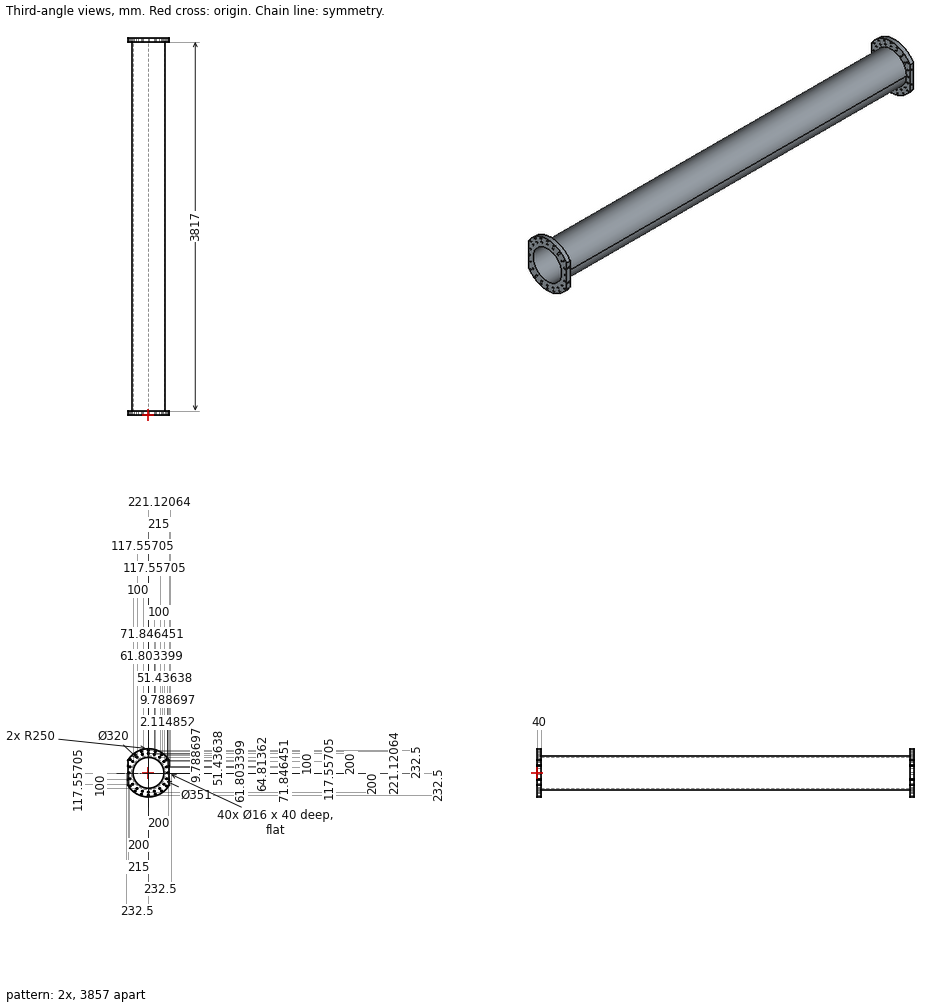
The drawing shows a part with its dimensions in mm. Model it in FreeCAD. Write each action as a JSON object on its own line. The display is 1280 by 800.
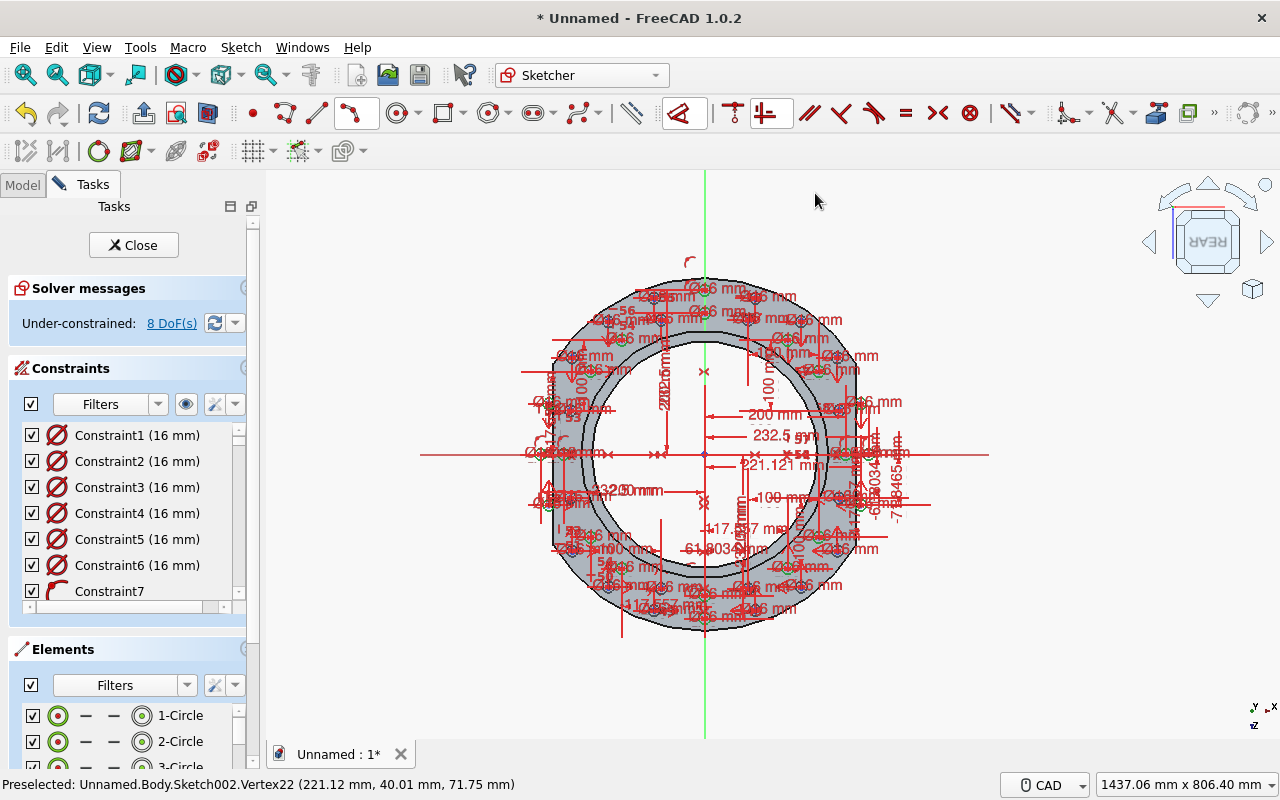
{"action": "left_click", "coordinate": [755, 611]}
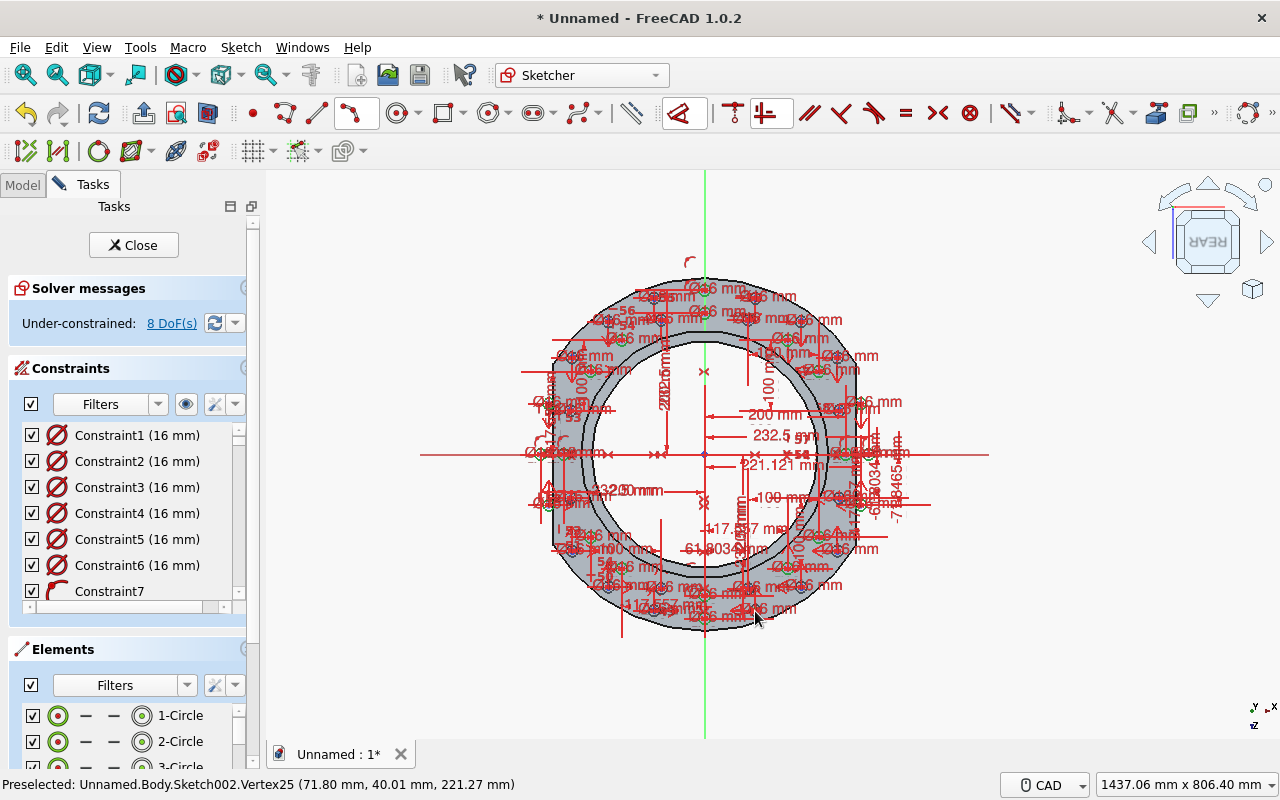
{"action": "left_click", "coordinate": [702, 114]}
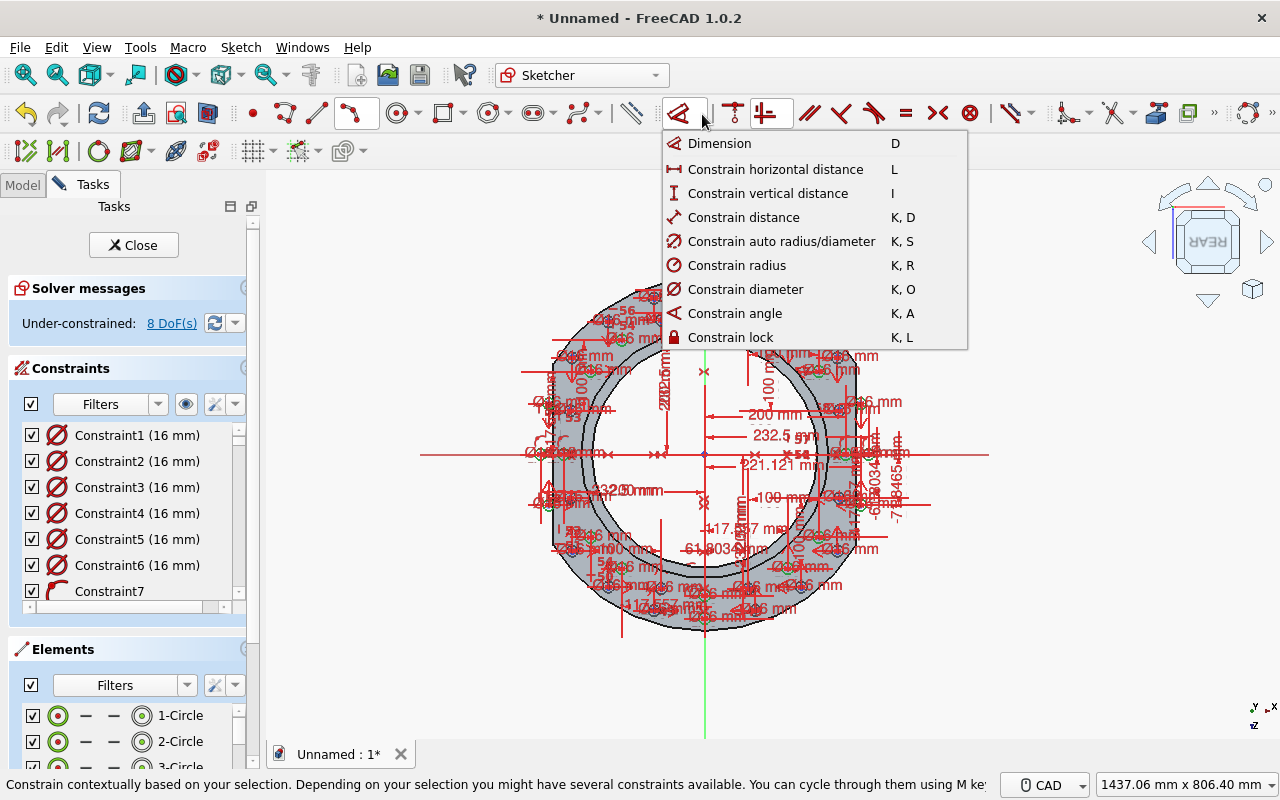
{"action": "left_click", "coordinate": [815, 169]}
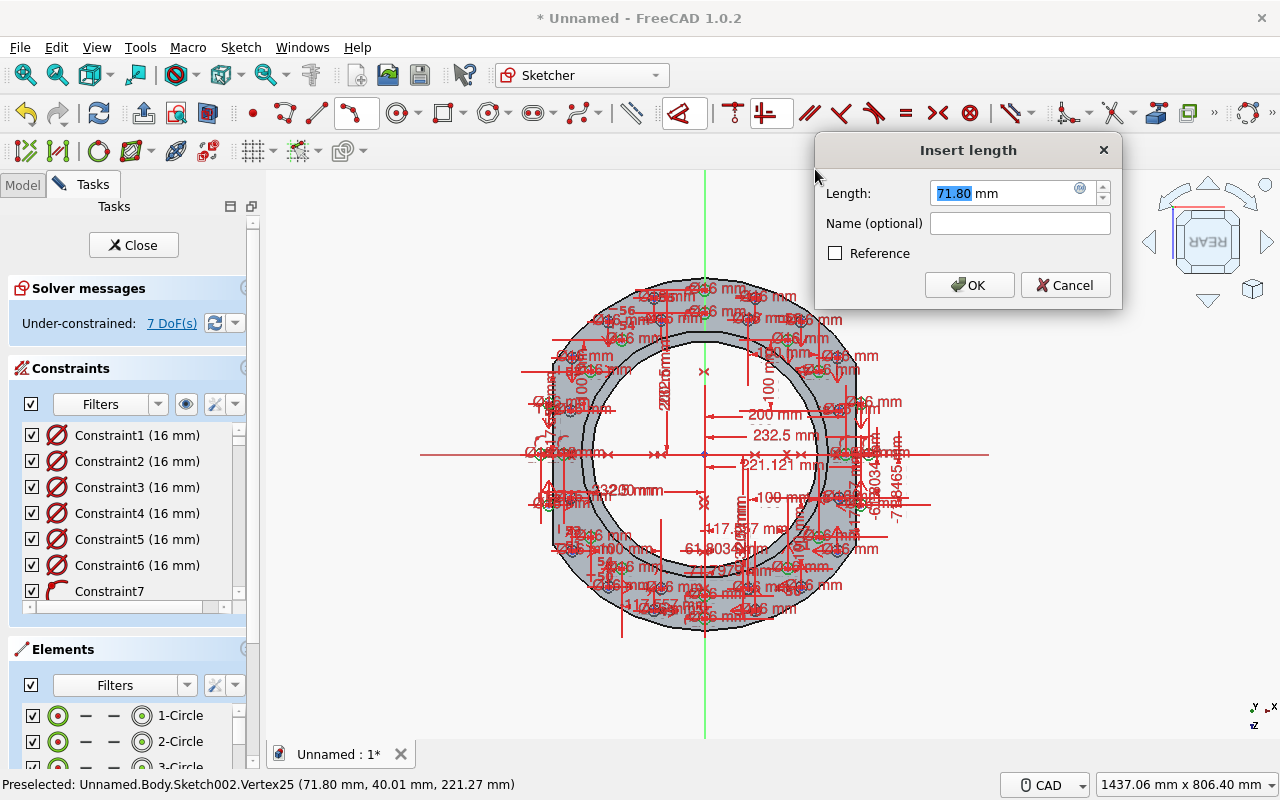
{"action": "type", "text": "71.846451"}
{"action": "key", "text": "Return"}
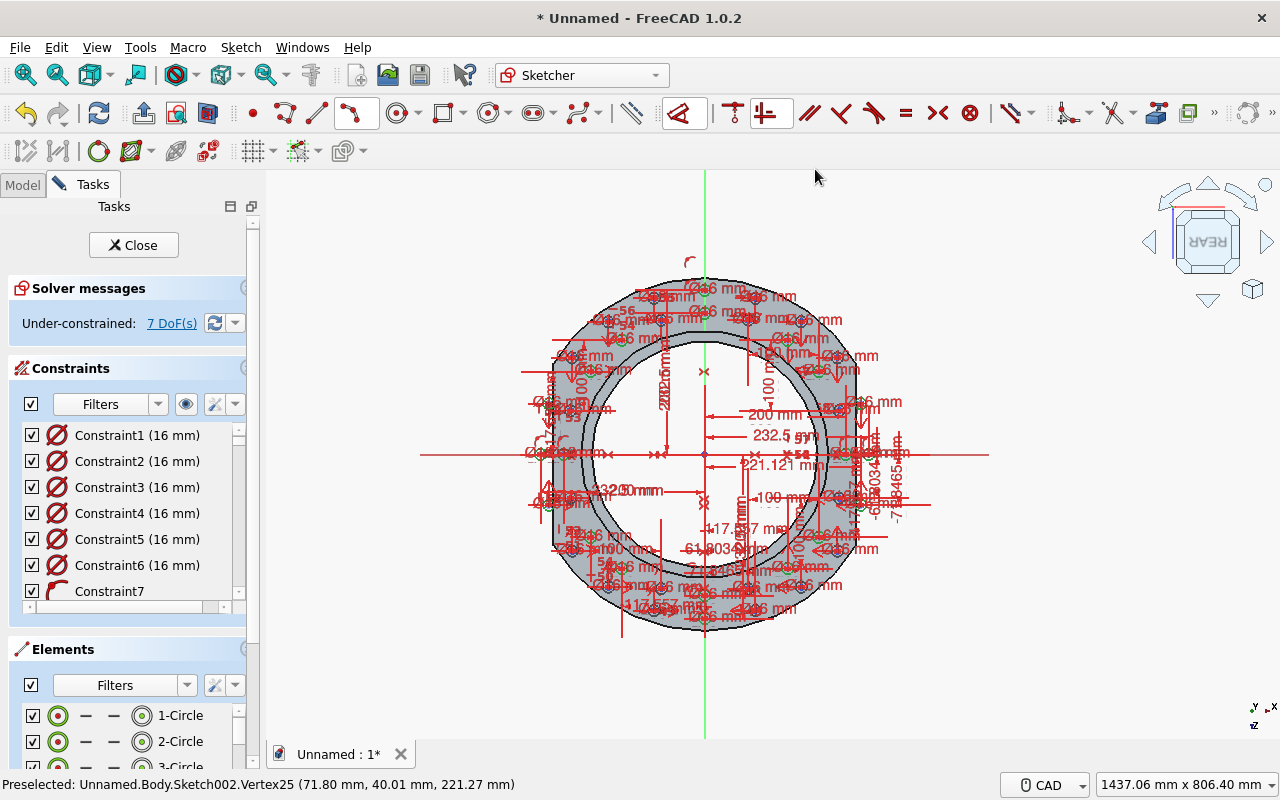
{"action": "left_click", "coordinate": [755, 611]}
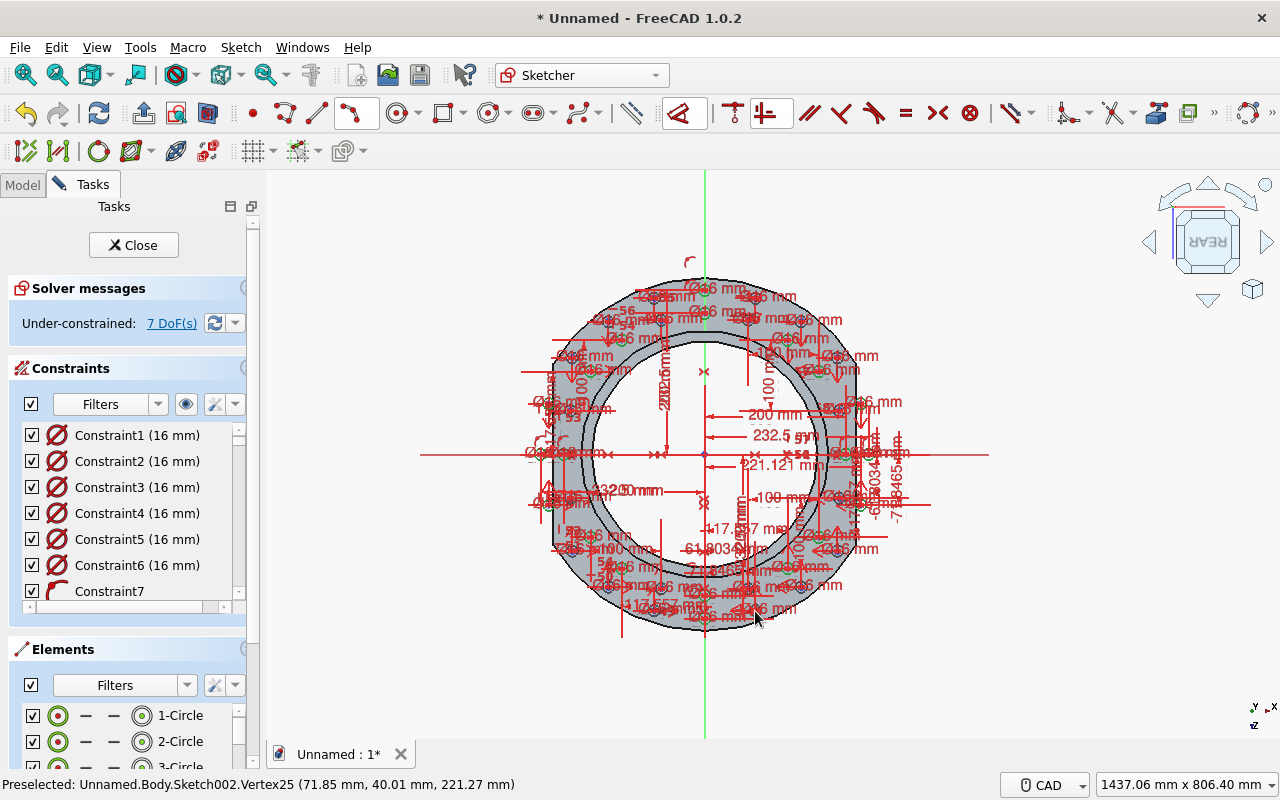
{"action": "left_click", "coordinate": [702, 114]}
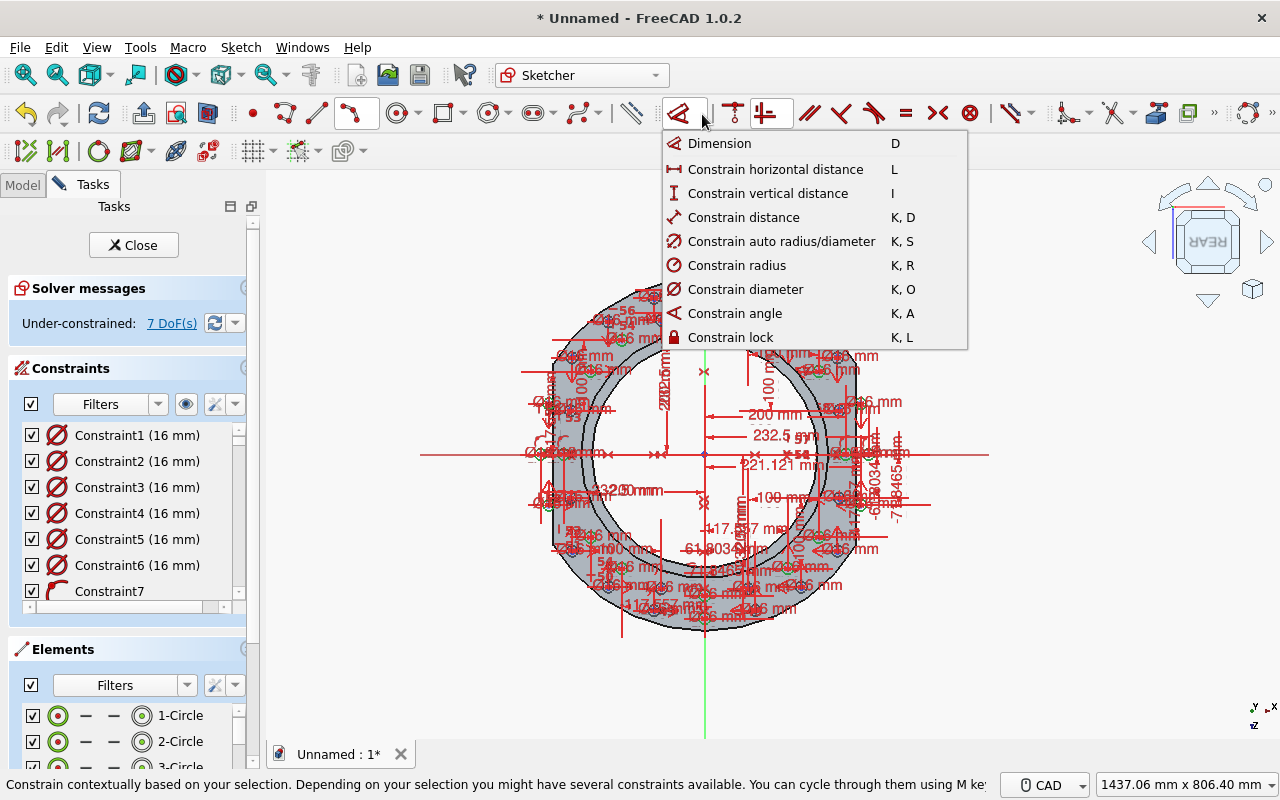
{"action": "left_click", "coordinate": [815, 193]}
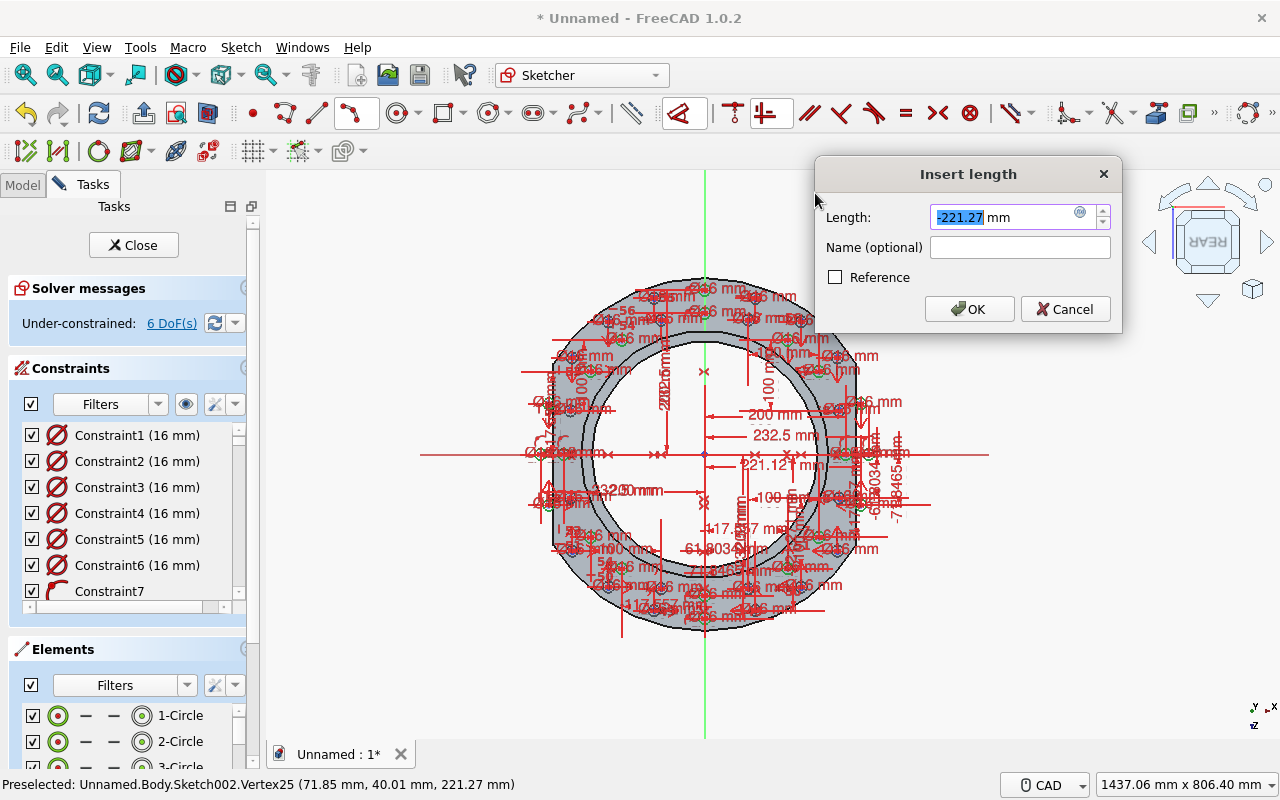
{"action": "type", "text": "-221.12064"}
{"action": "key", "text": "Return"}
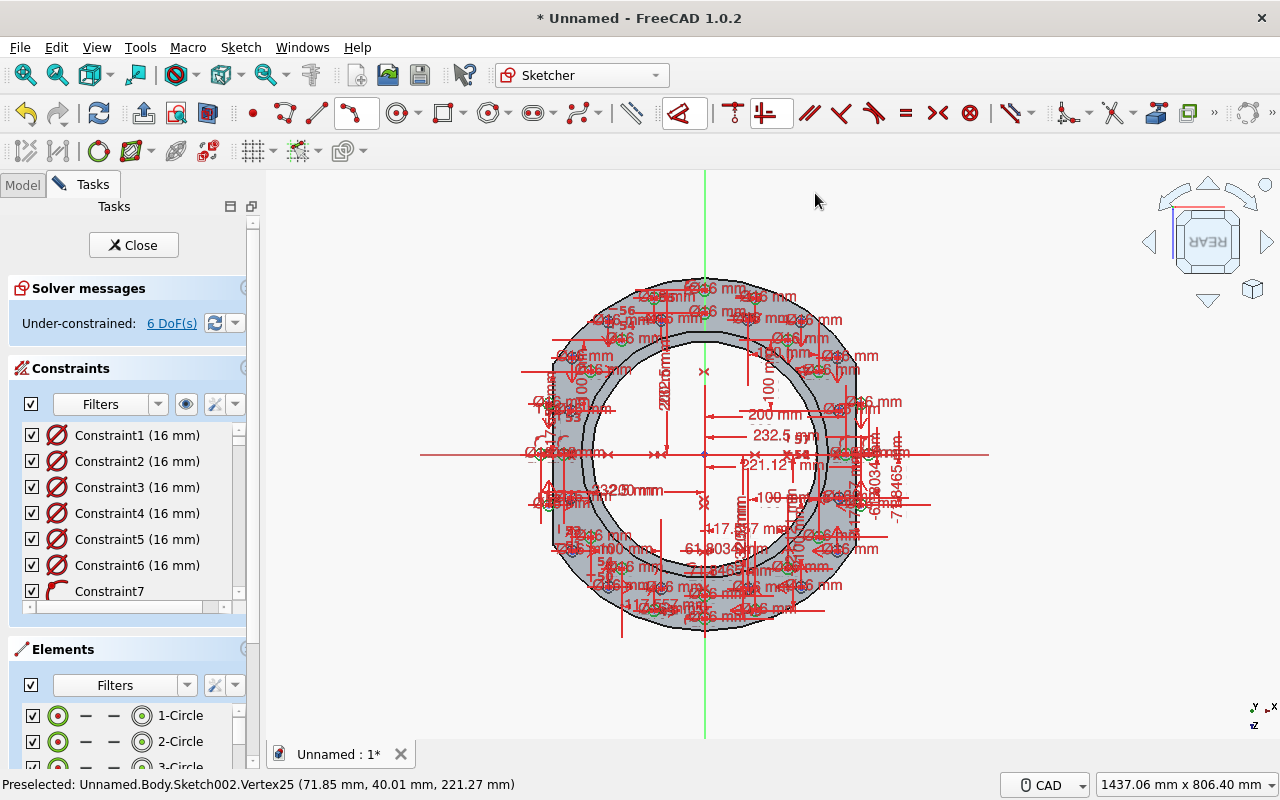
{"action": "scroll", "coordinate": [846, 454], "scroll_direction": "up", "scroll_amount": 9}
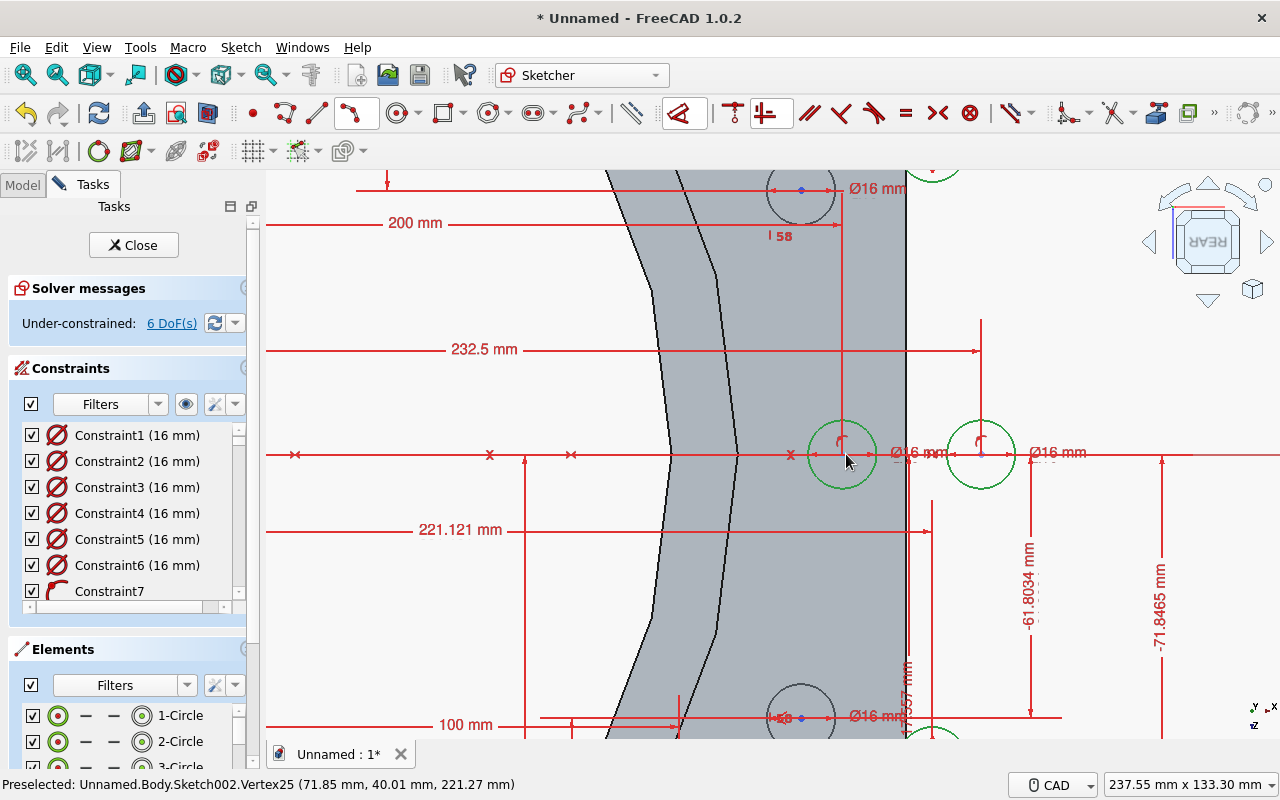
{"action": "left_click", "coordinate": [842, 454]}